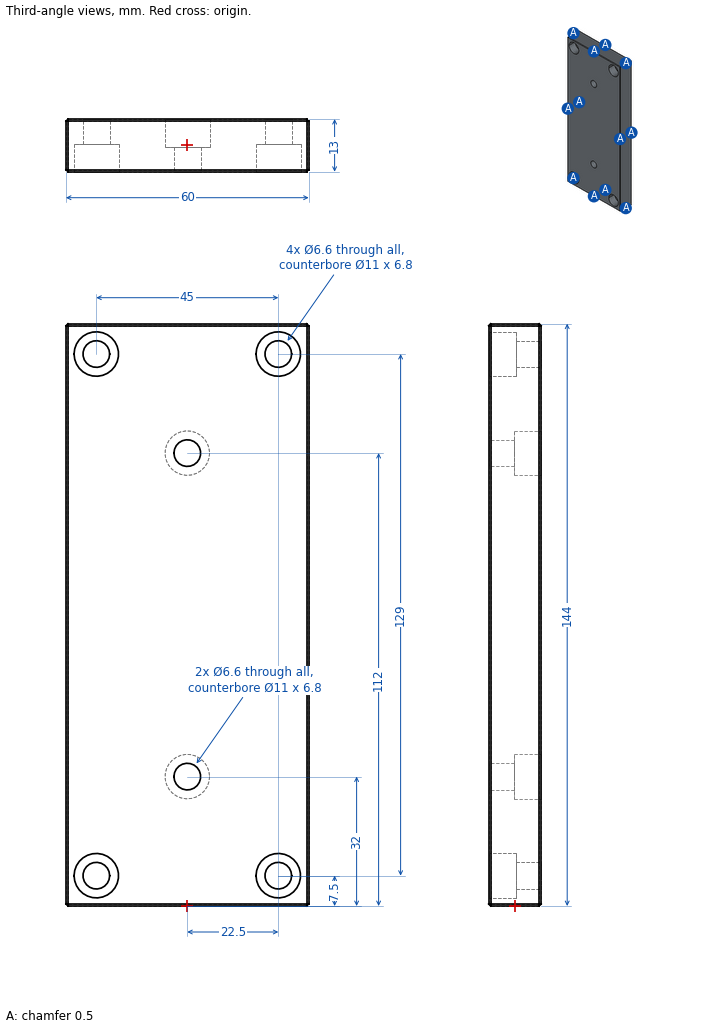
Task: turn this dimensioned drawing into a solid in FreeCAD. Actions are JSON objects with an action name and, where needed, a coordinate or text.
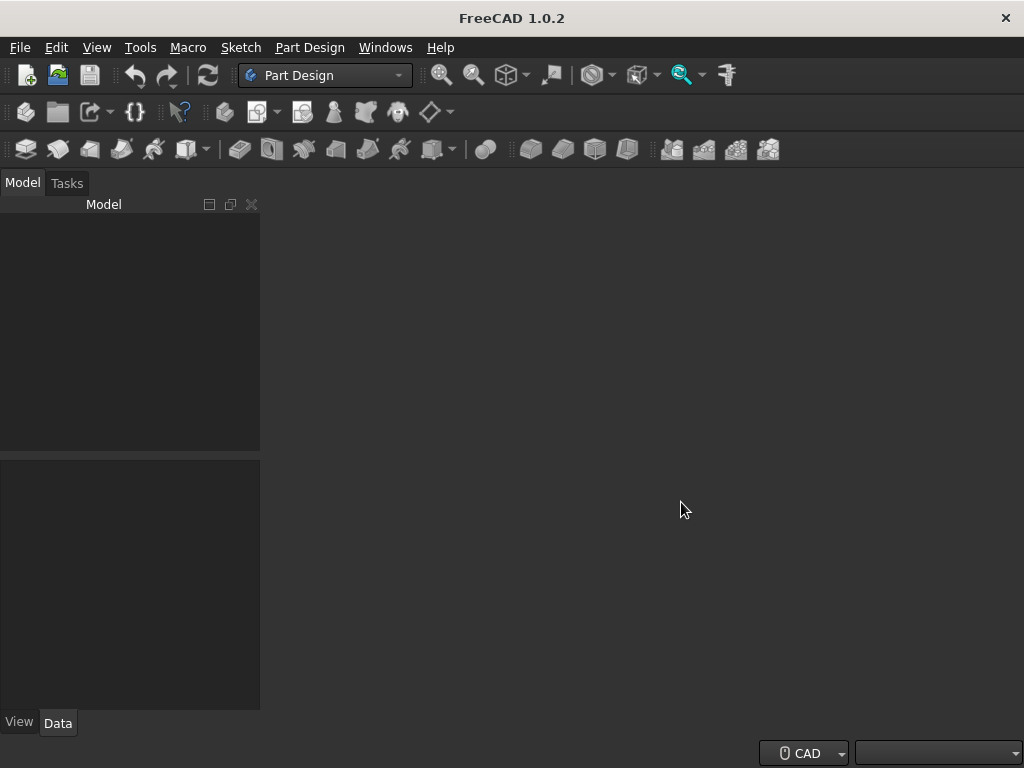
{"action": "key", "text": "ctrl+n"}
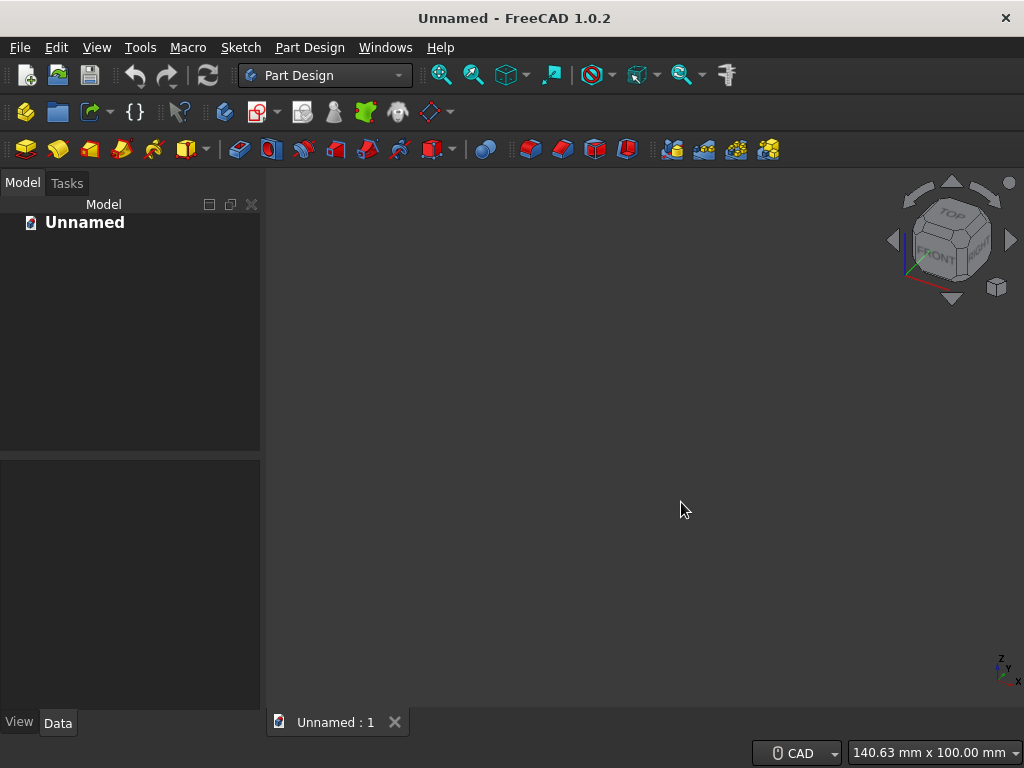
{"action": "left_click", "coordinate": [258, 112]}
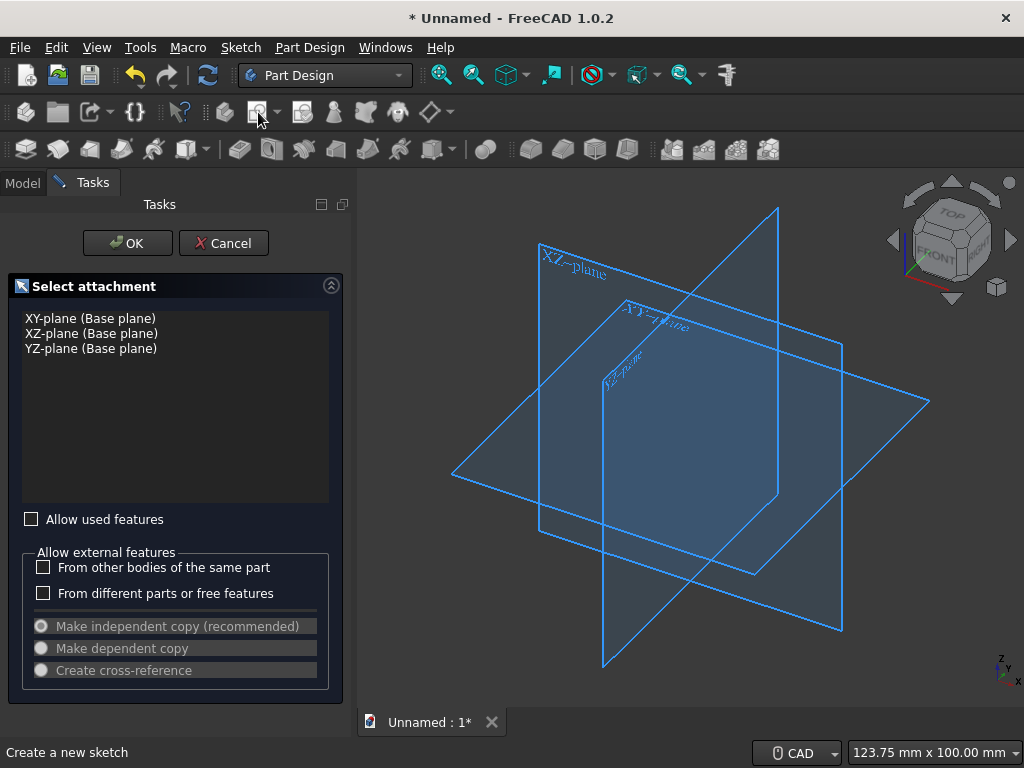
{"action": "left_click", "coordinate": [82, 318]}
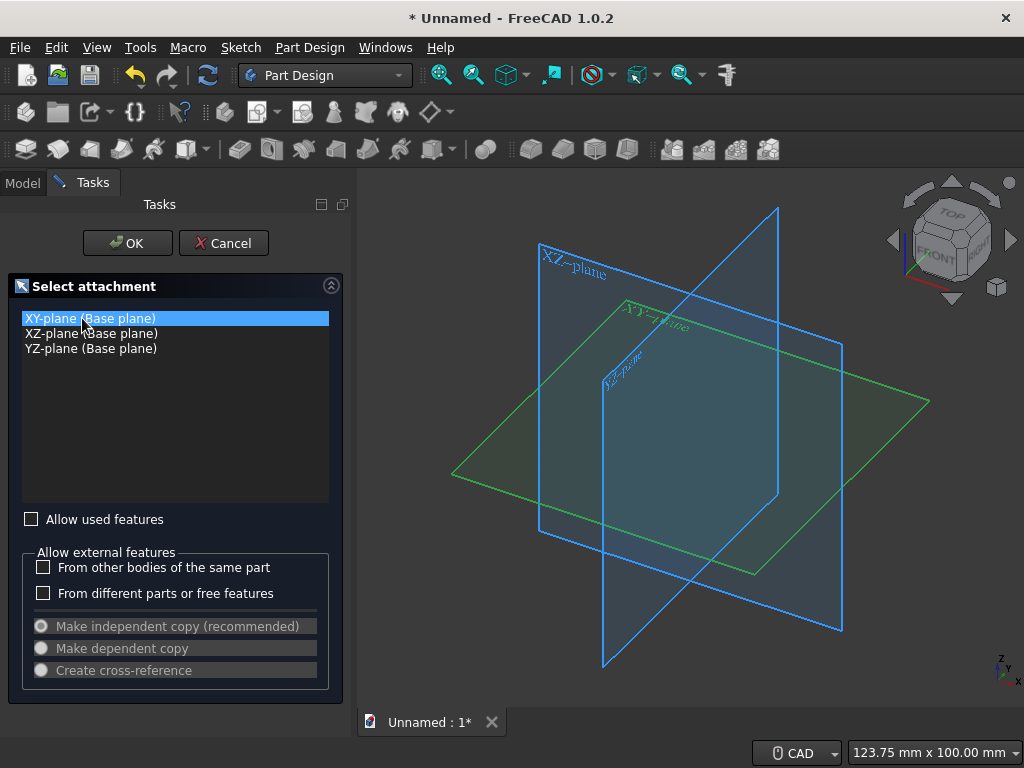
{"action": "left_click", "coordinate": [128, 243]}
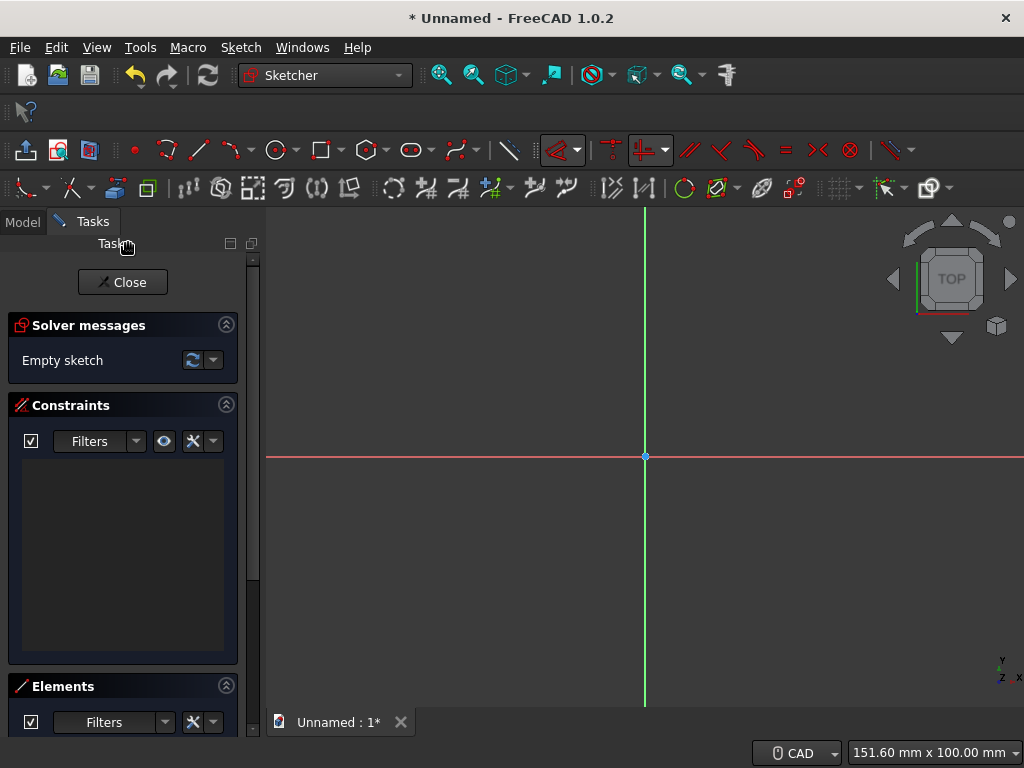
{"action": "key", "text": "g v"}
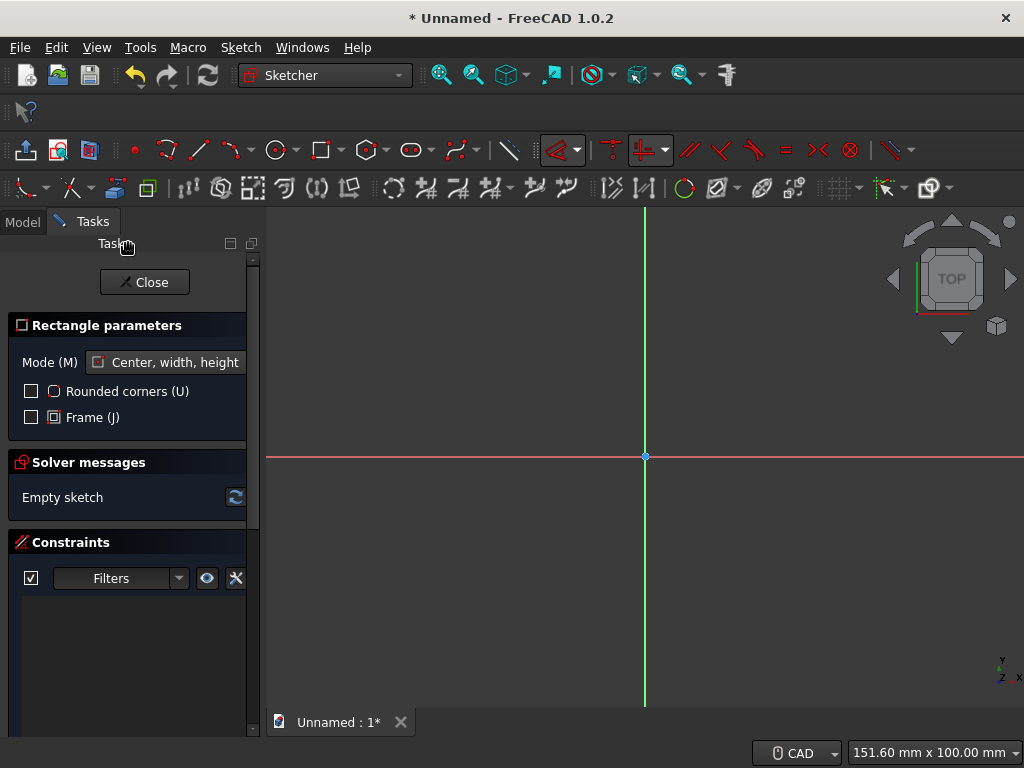
{"action": "left_click", "coordinate": [645, 457]}
{"action": "left_click", "coordinate": [795, 424]}
{"action": "key", "text": "Escape"}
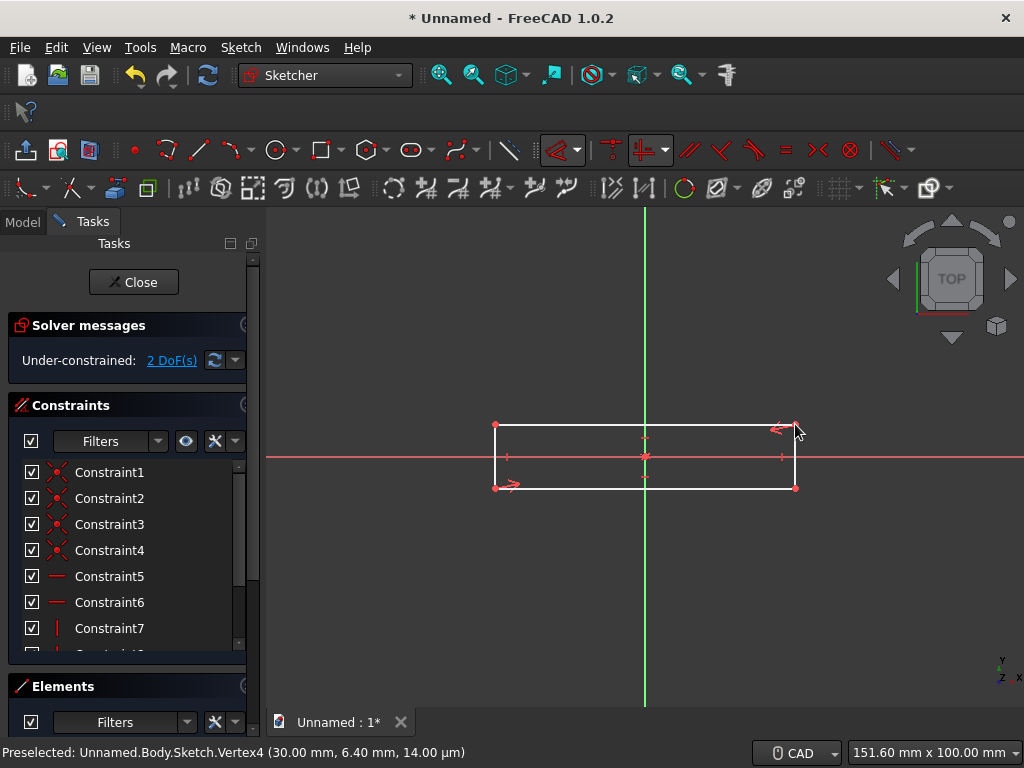
{"action": "left_click", "coordinate": [585, 489]}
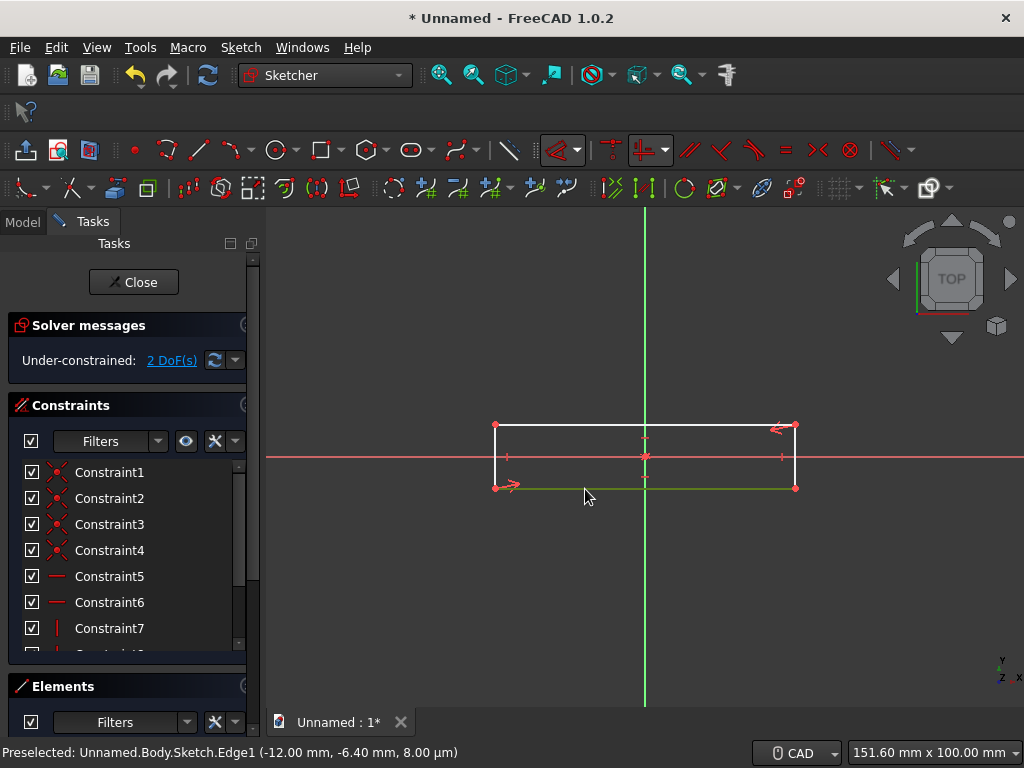
{"action": "key", "text": "l"}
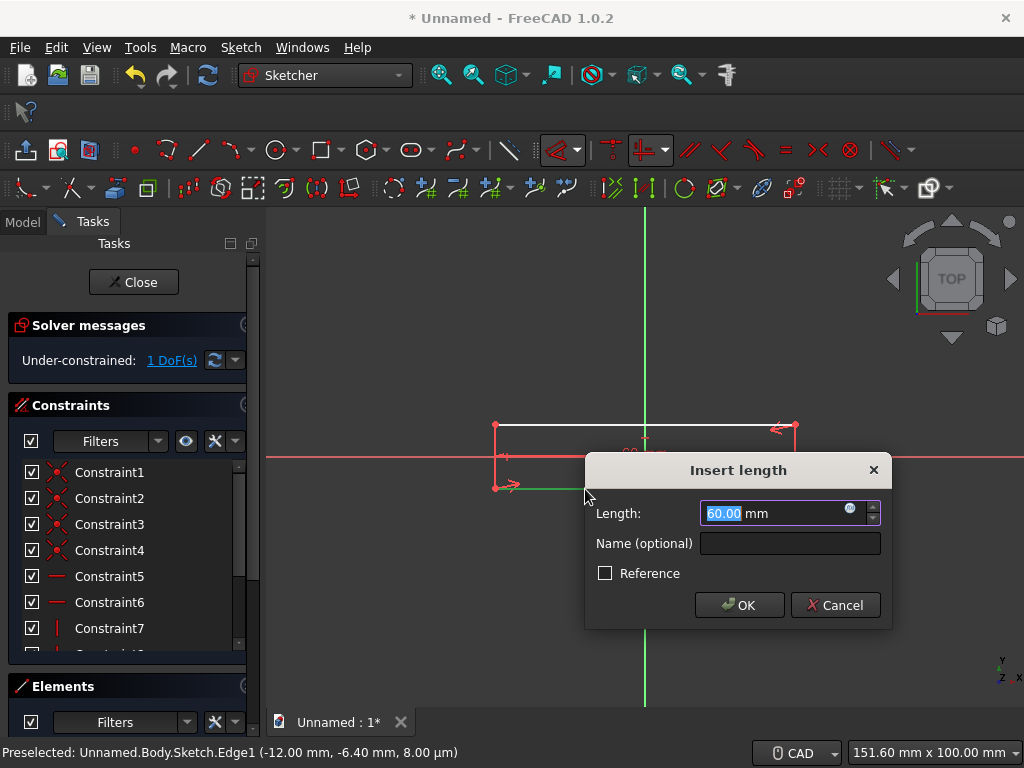
{"action": "type", "text": "60"}
{"action": "key", "text": "Return"}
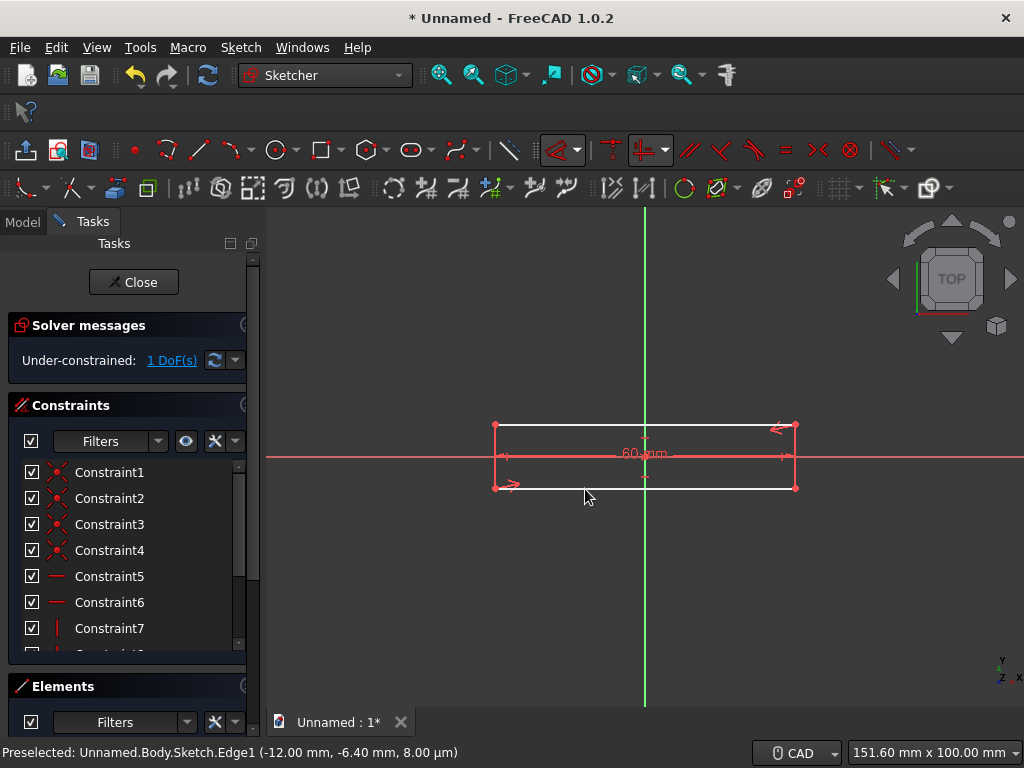
{"action": "left_click", "coordinate": [795, 470]}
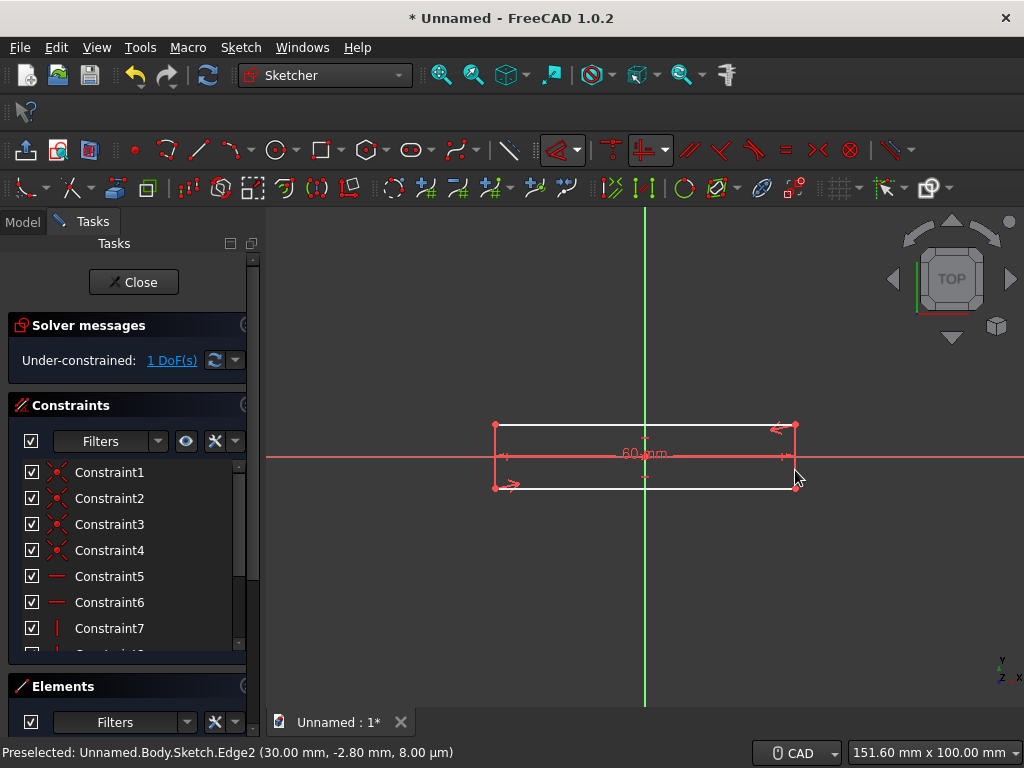
{"action": "key", "text": "i"}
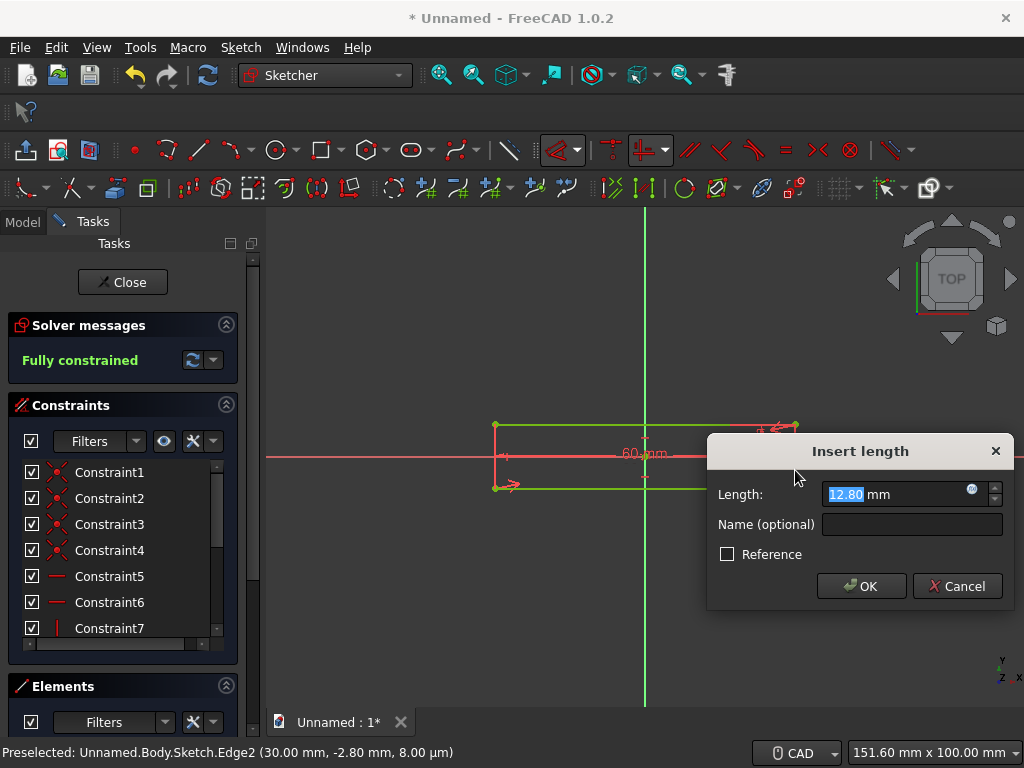
{"action": "type", "text": "13"}
{"action": "key", "text": "Return"}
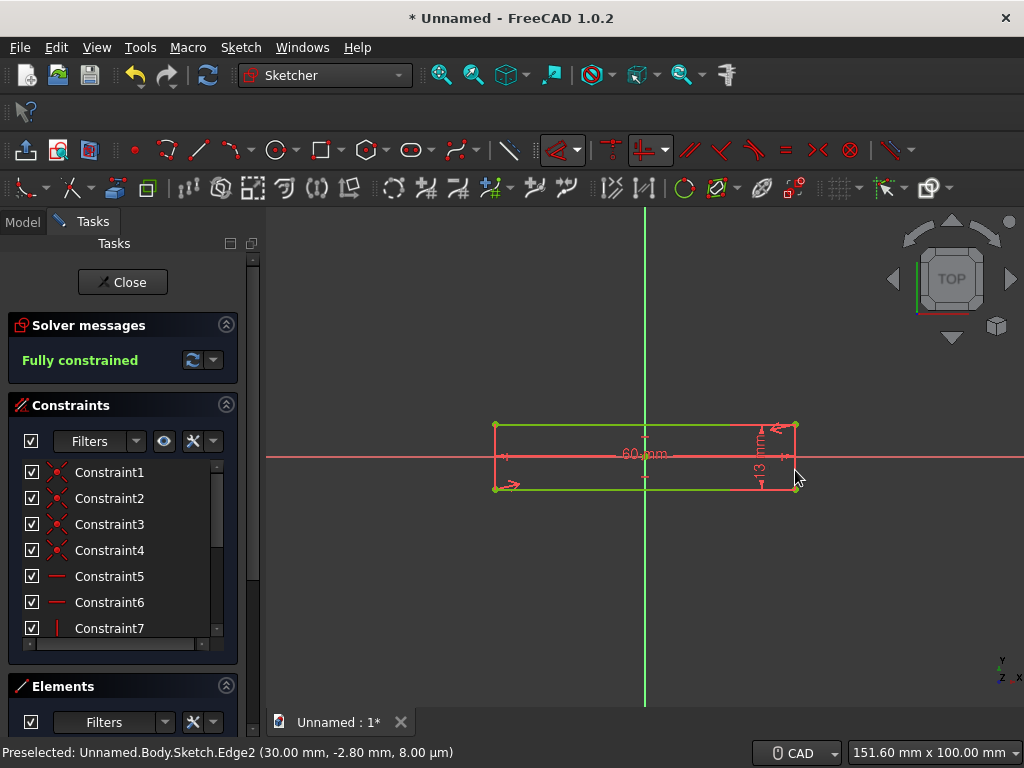
{"action": "left_click", "coordinate": [123, 282]}